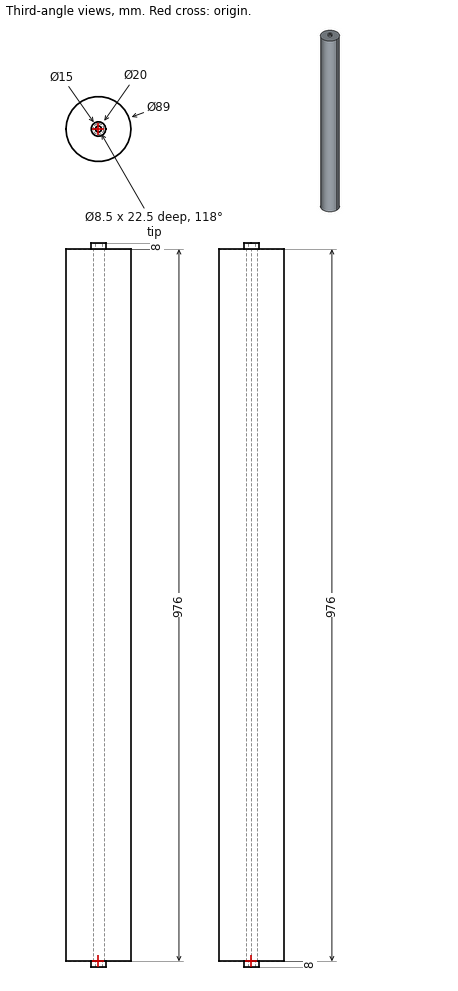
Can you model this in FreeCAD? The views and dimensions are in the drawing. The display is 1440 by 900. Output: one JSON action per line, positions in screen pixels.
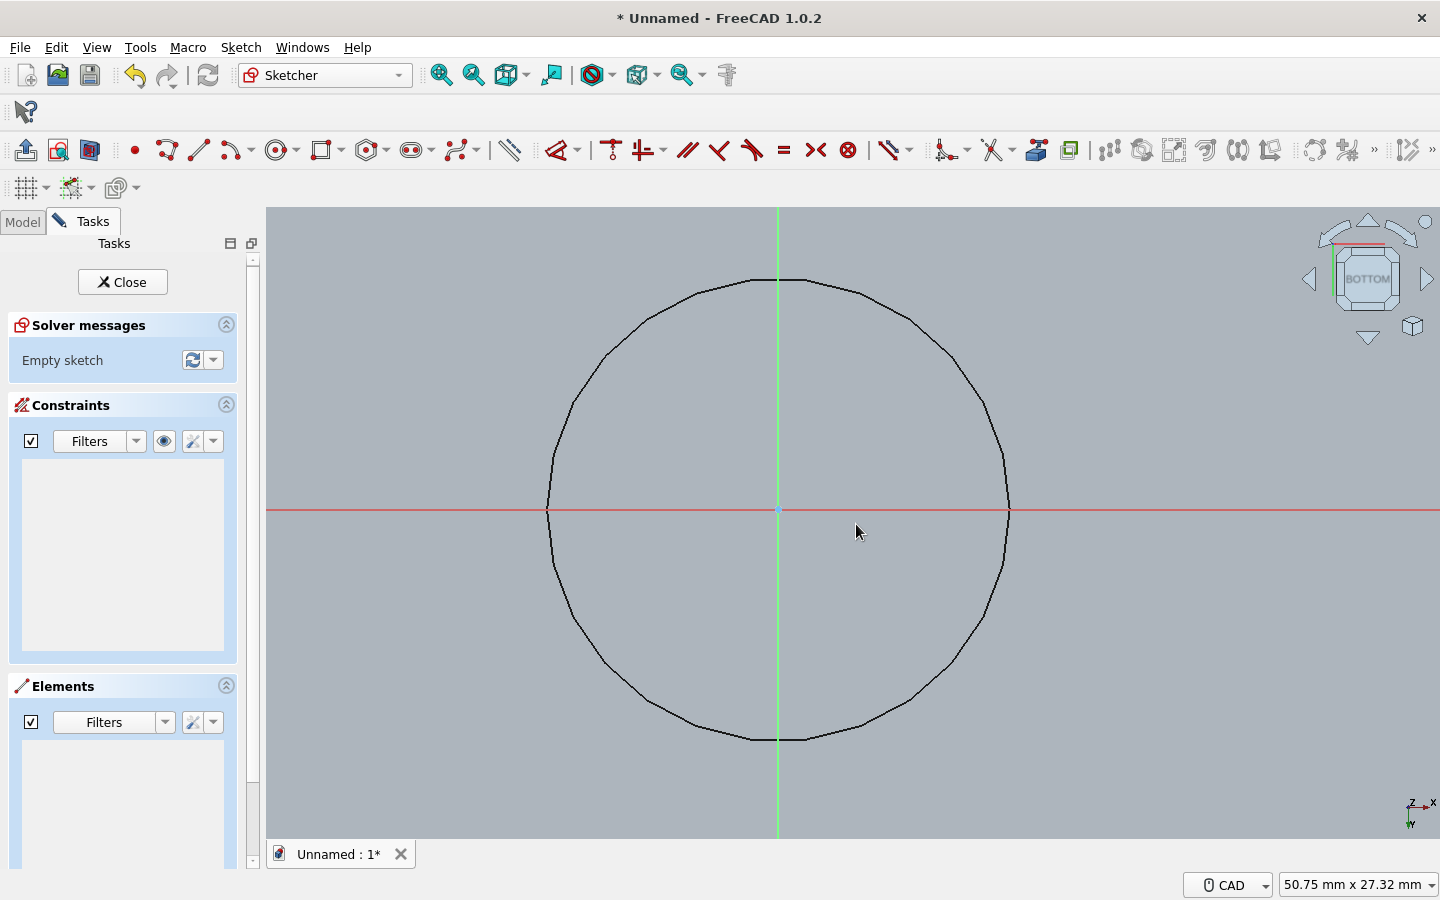
{"action": "scroll", "coordinate": [773, 499], "scroll_direction": "up", "scroll_amount": 4}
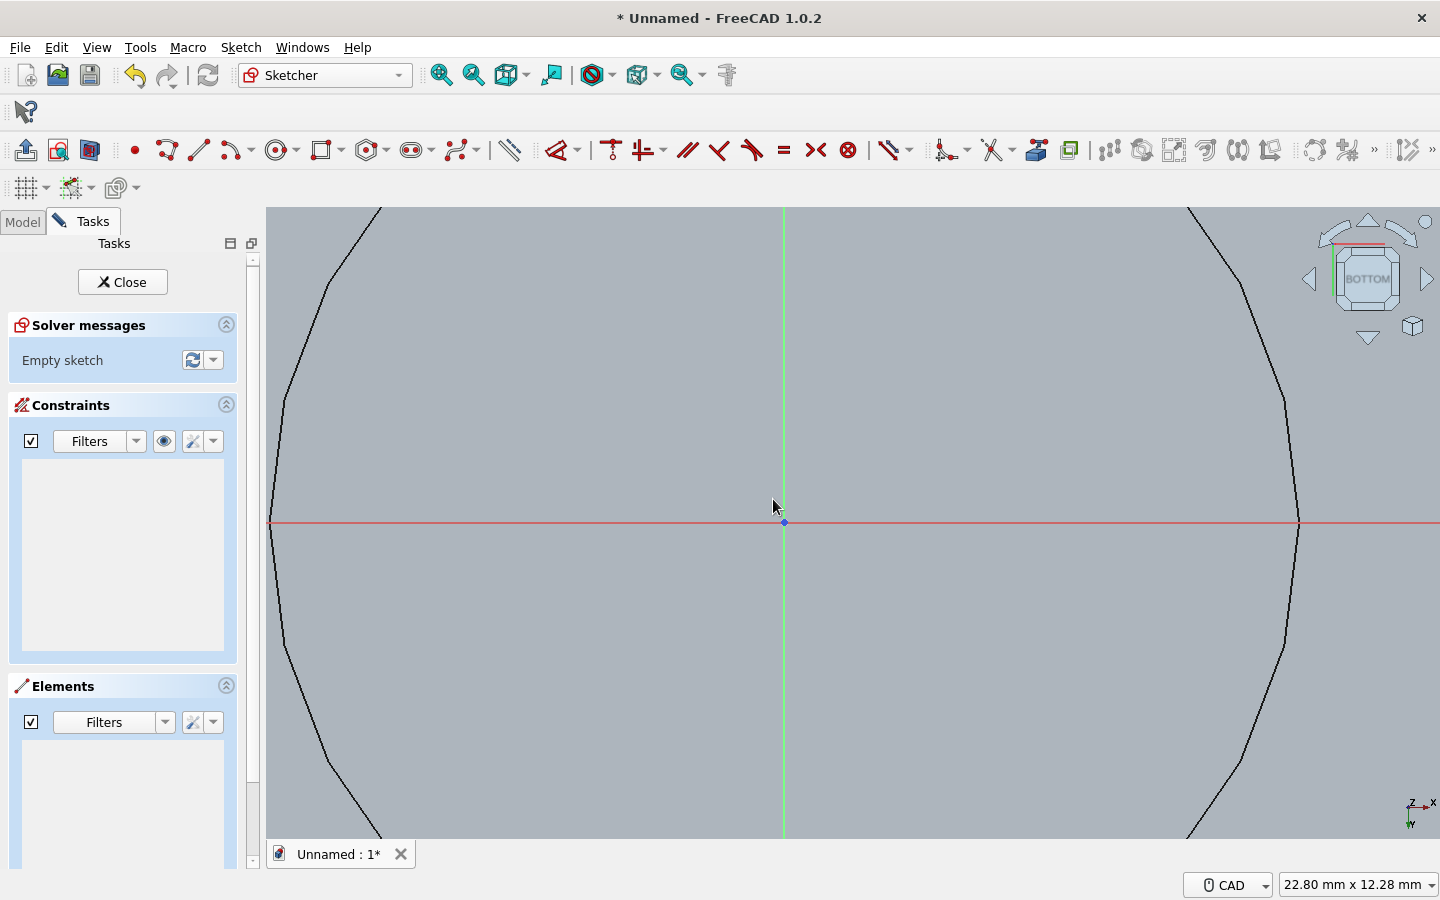
{"action": "left_click", "coordinate": [276, 150]}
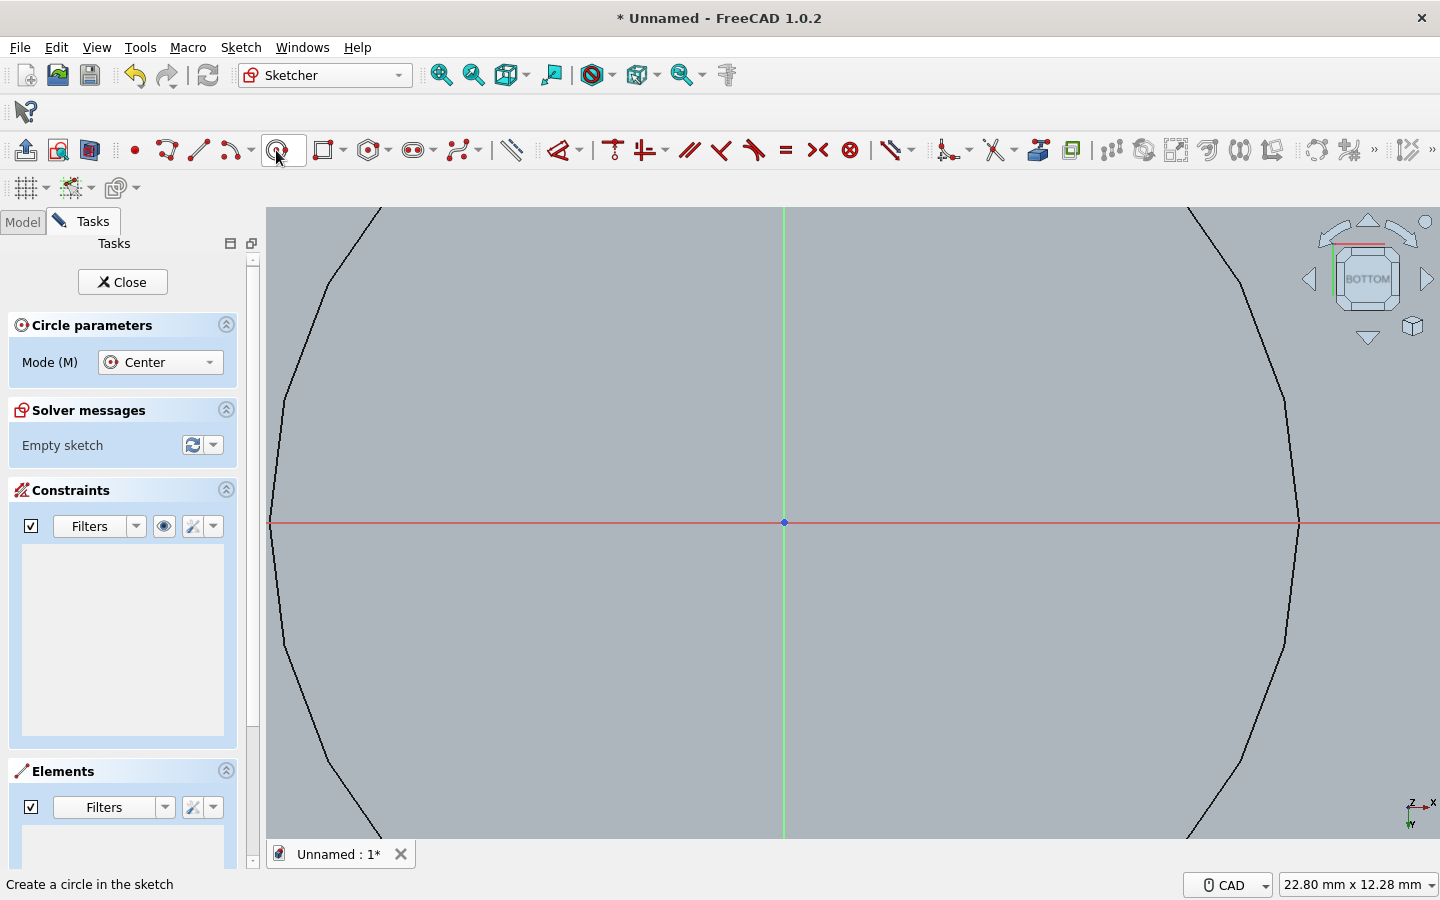
{"action": "left_click", "coordinate": [784, 523]}
{"action": "left_click", "coordinate": [939, 368]}
{"action": "key", "text": "Escape"}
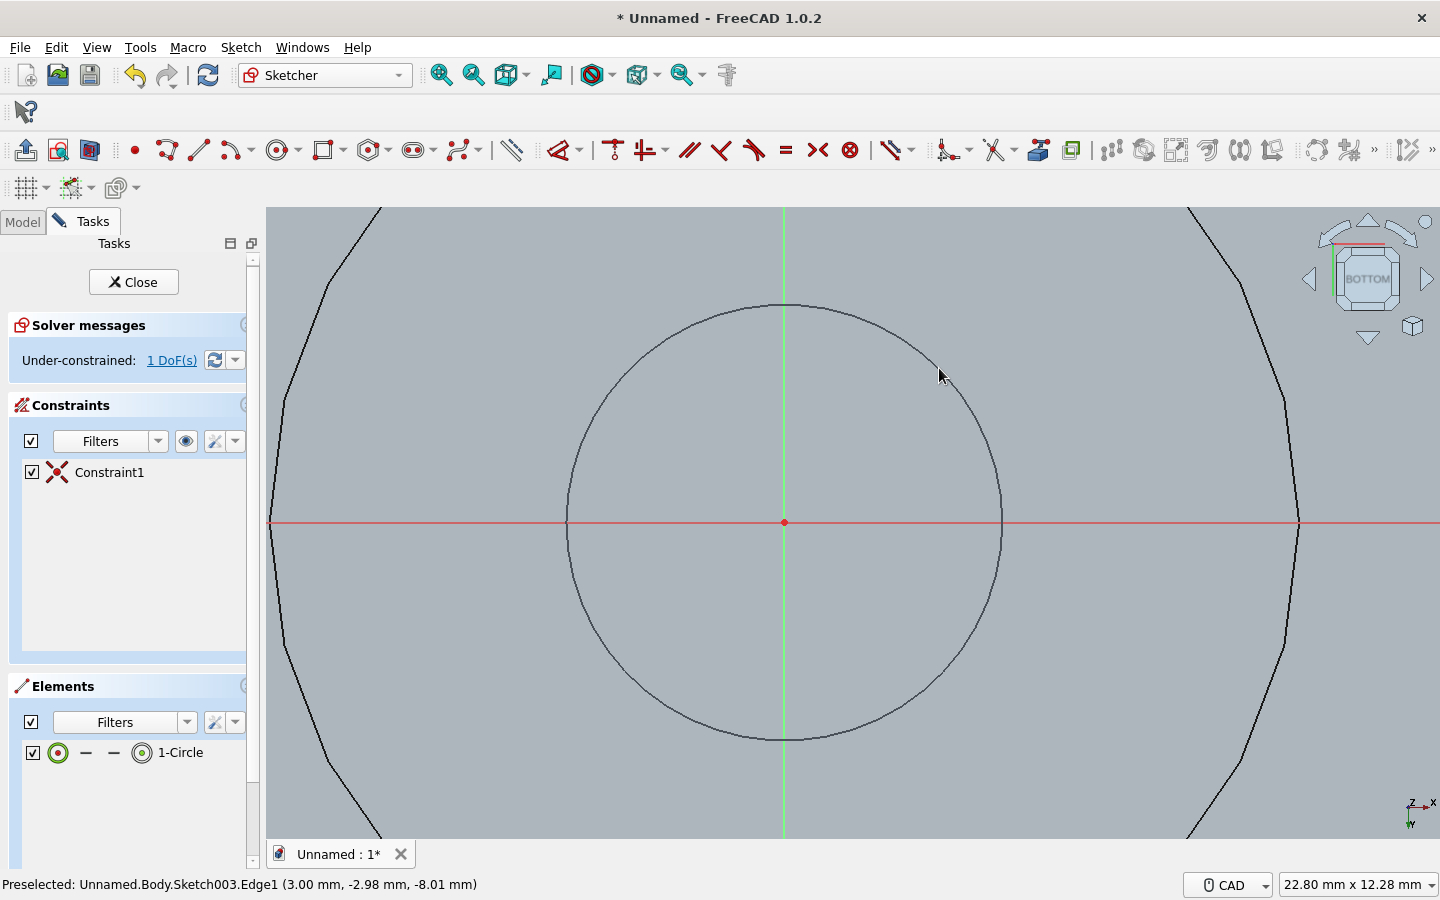
{"action": "left_click", "coordinate": [558, 150]}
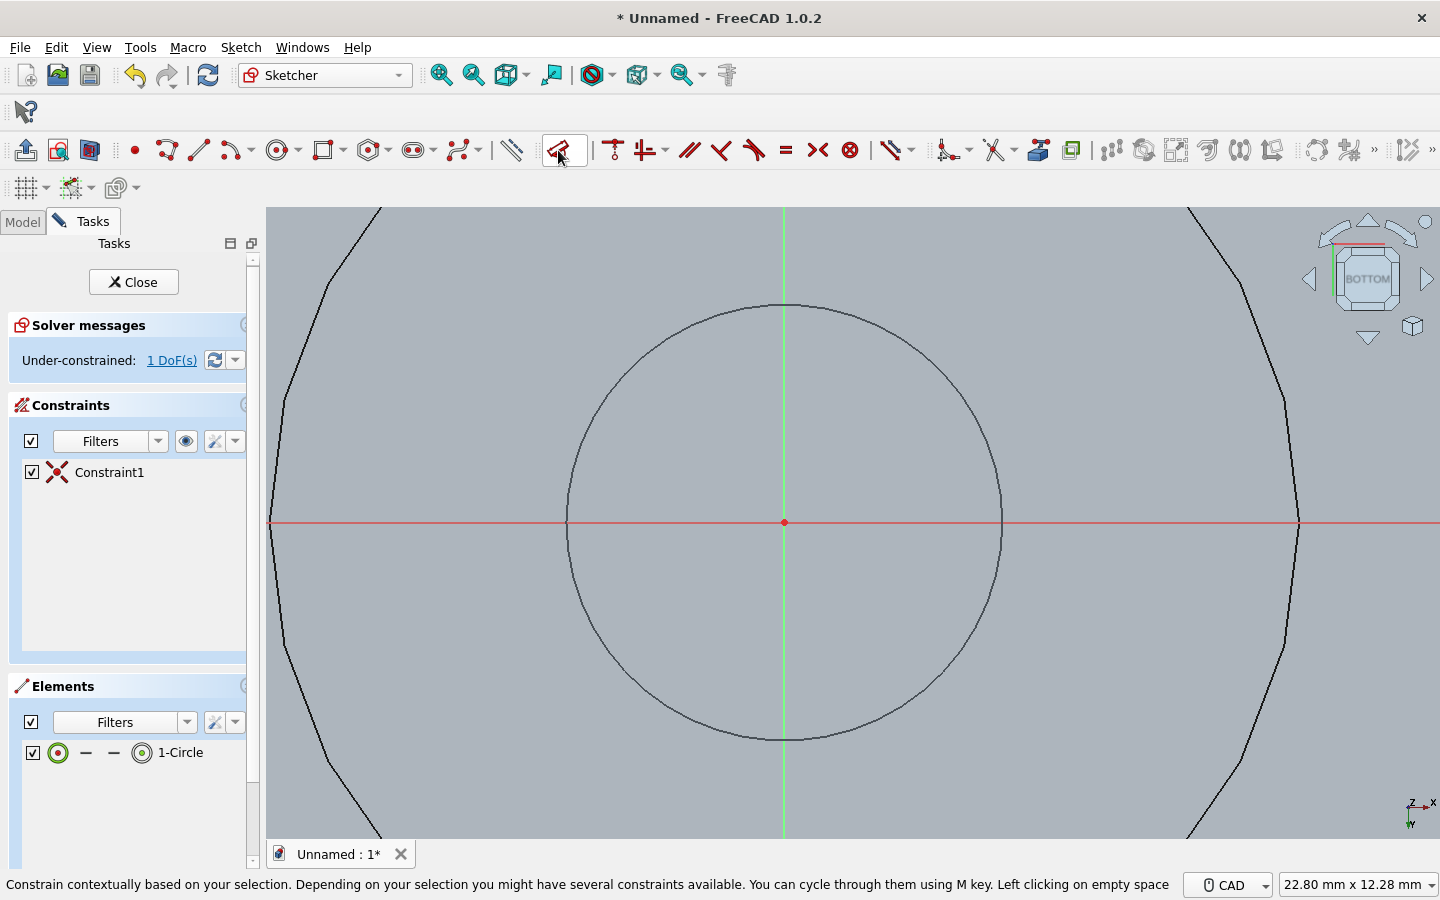
{"action": "left_click", "coordinate": [938, 368]}
{"action": "left_click", "coordinate": [961, 345]}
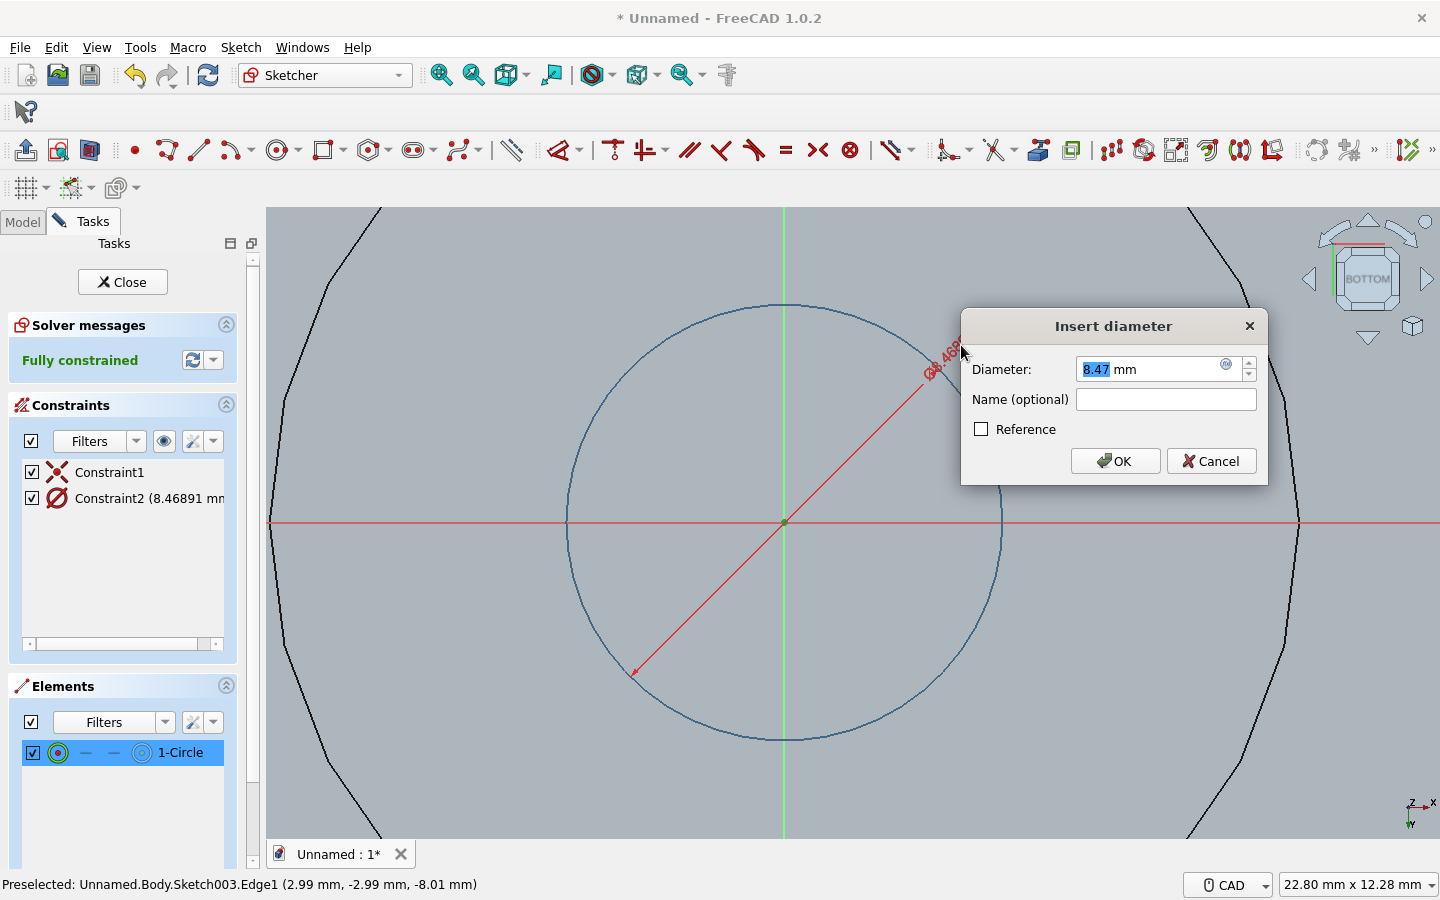
{"action": "type", "text": "8.5"}
{"action": "key", "text": "Return"}
{"action": "key", "text": "Escape"}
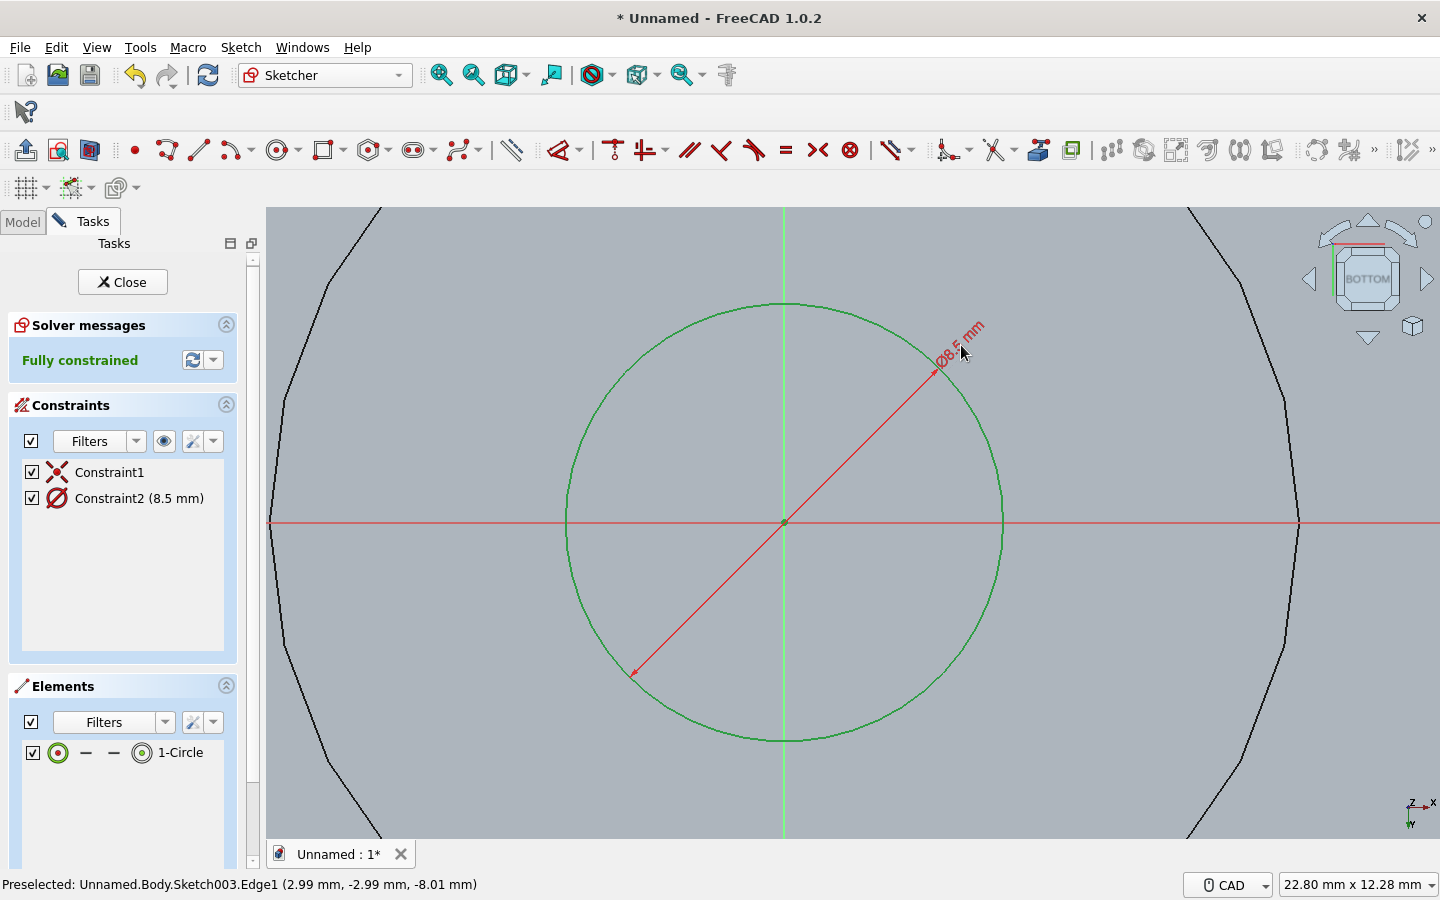
{"action": "left_click", "coordinate": [123, 282]}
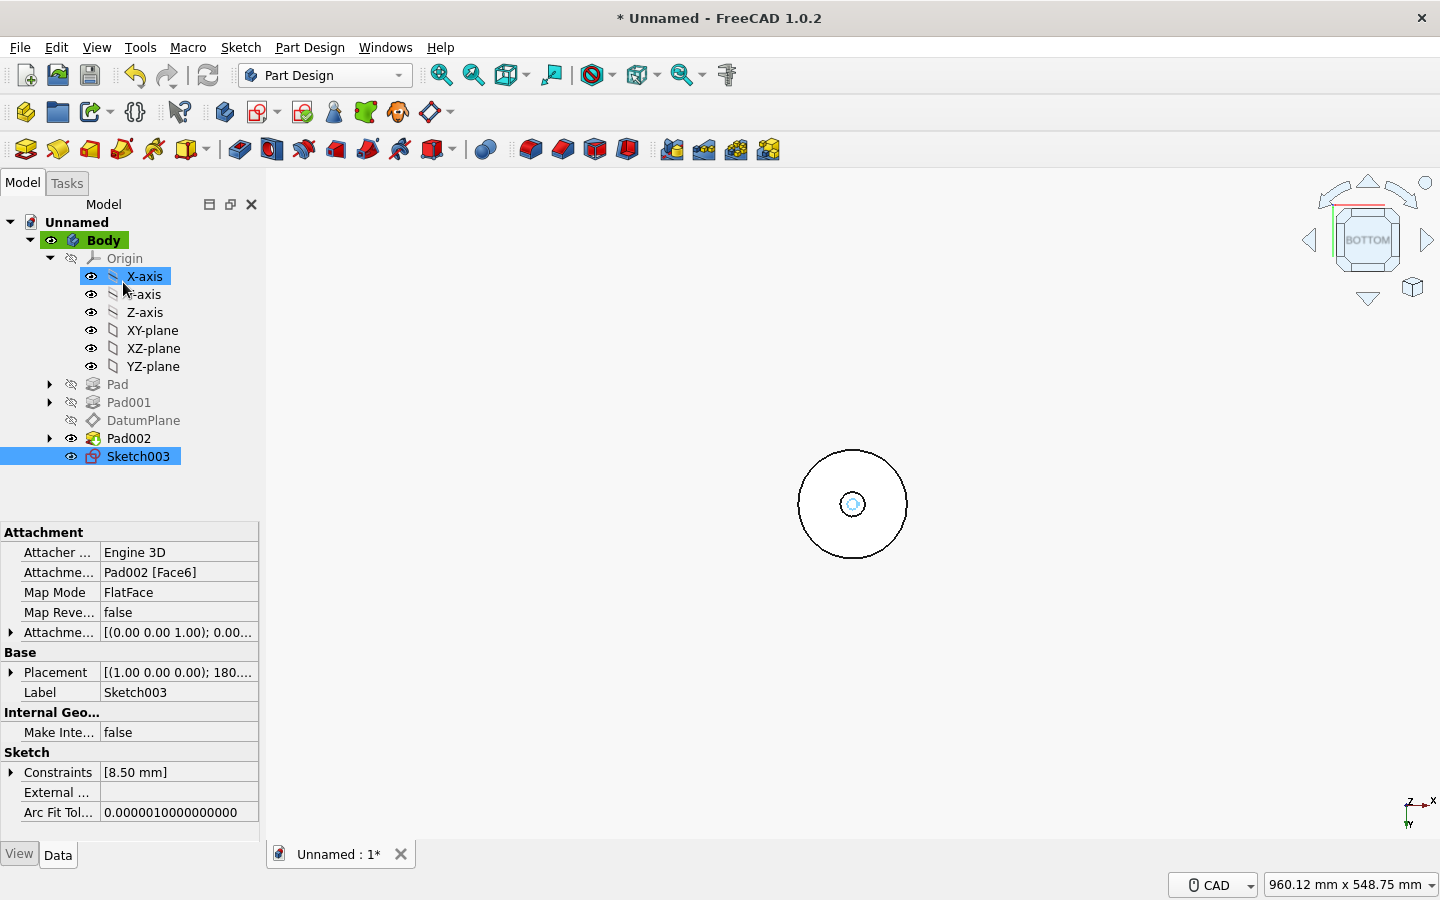
{"action": "left_click", "coordinate": [272, 150]}